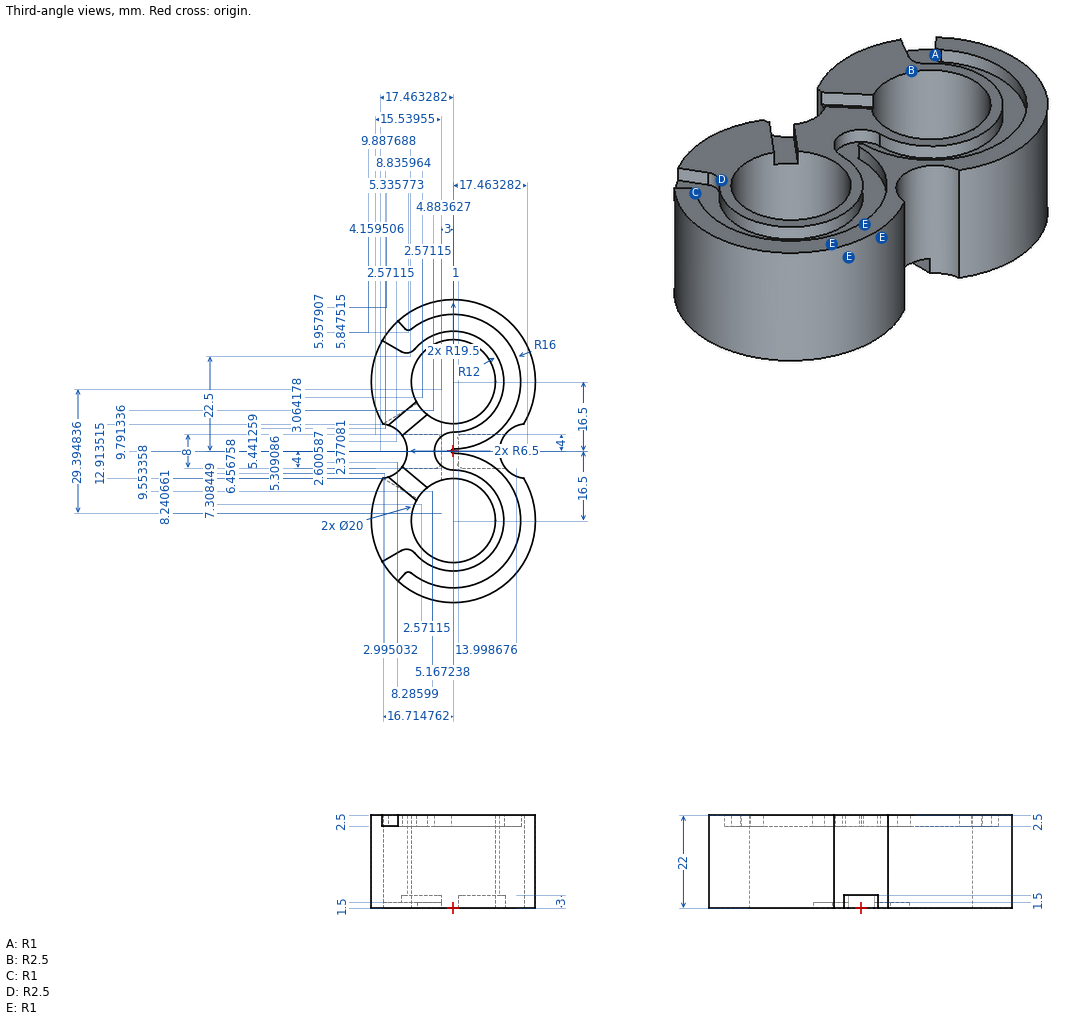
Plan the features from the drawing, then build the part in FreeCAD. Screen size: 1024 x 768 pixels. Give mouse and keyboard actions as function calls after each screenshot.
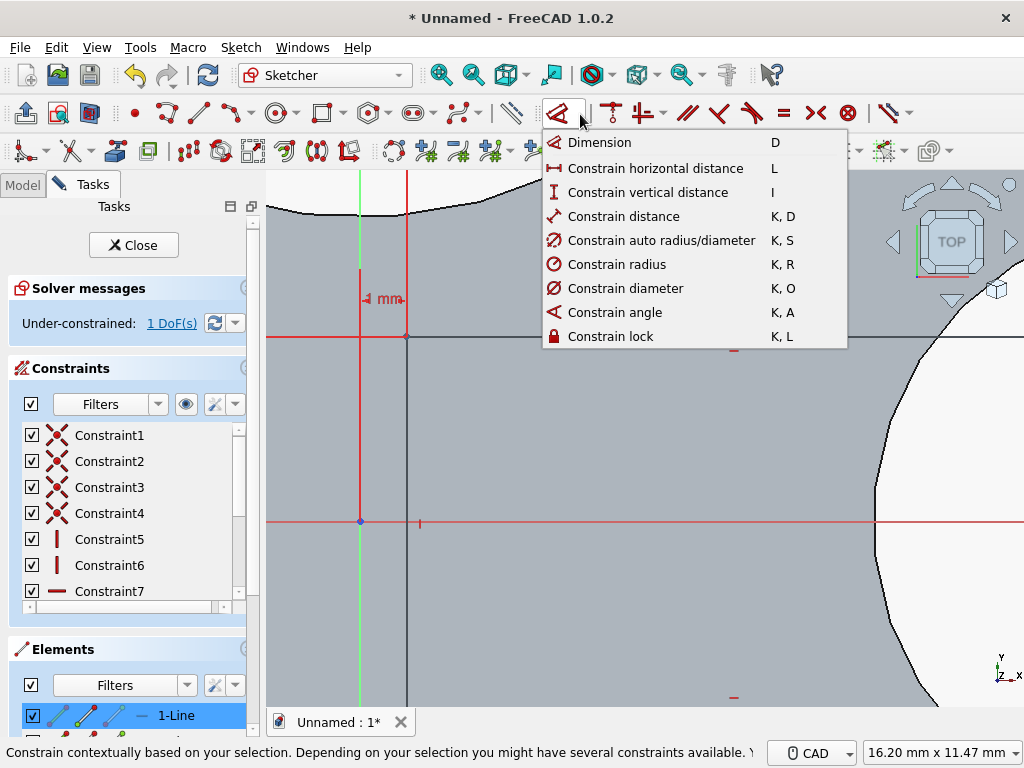
click(695, 192)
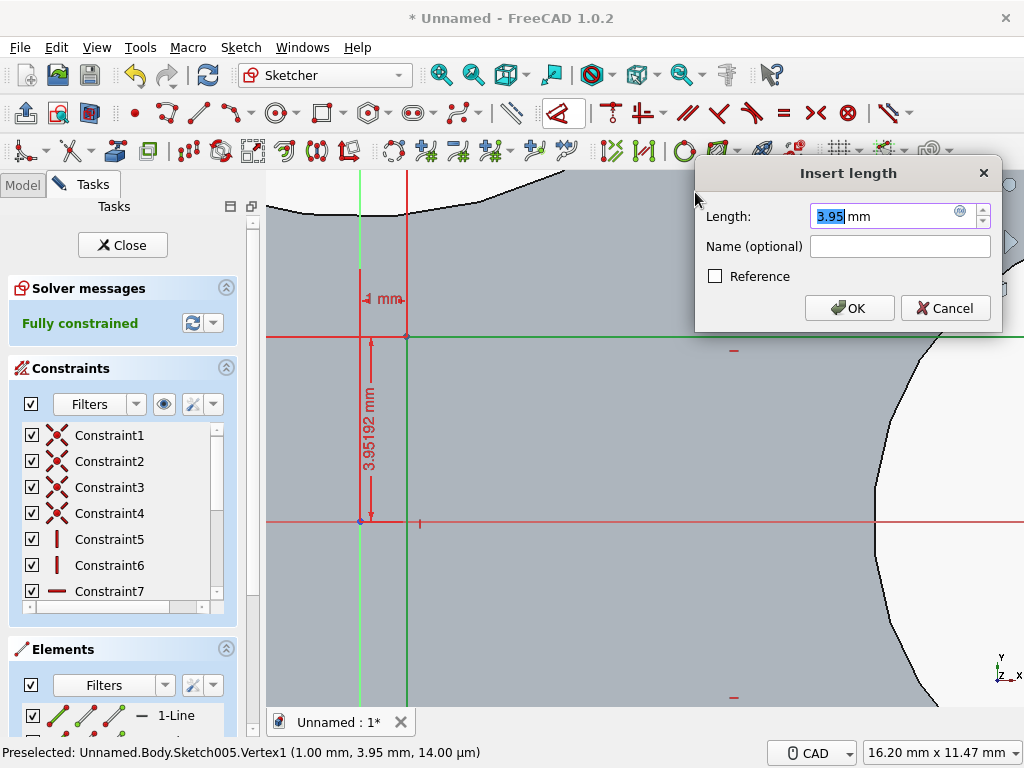
text(4)
key(Return)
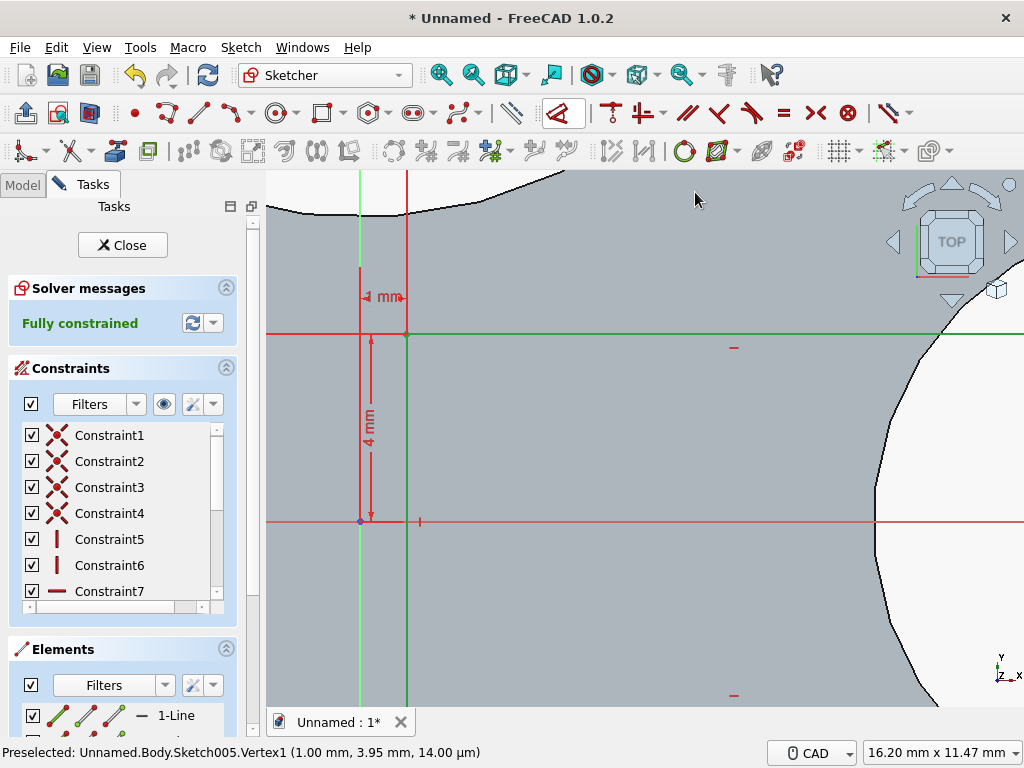
click(123, 245)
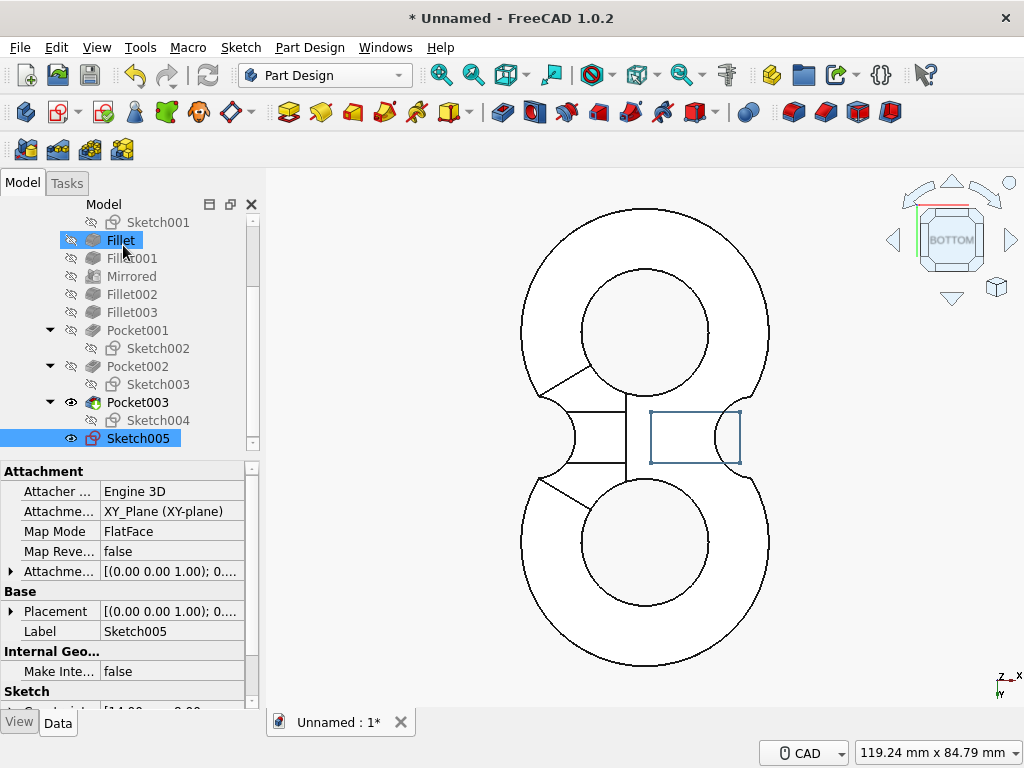
click(504, 112)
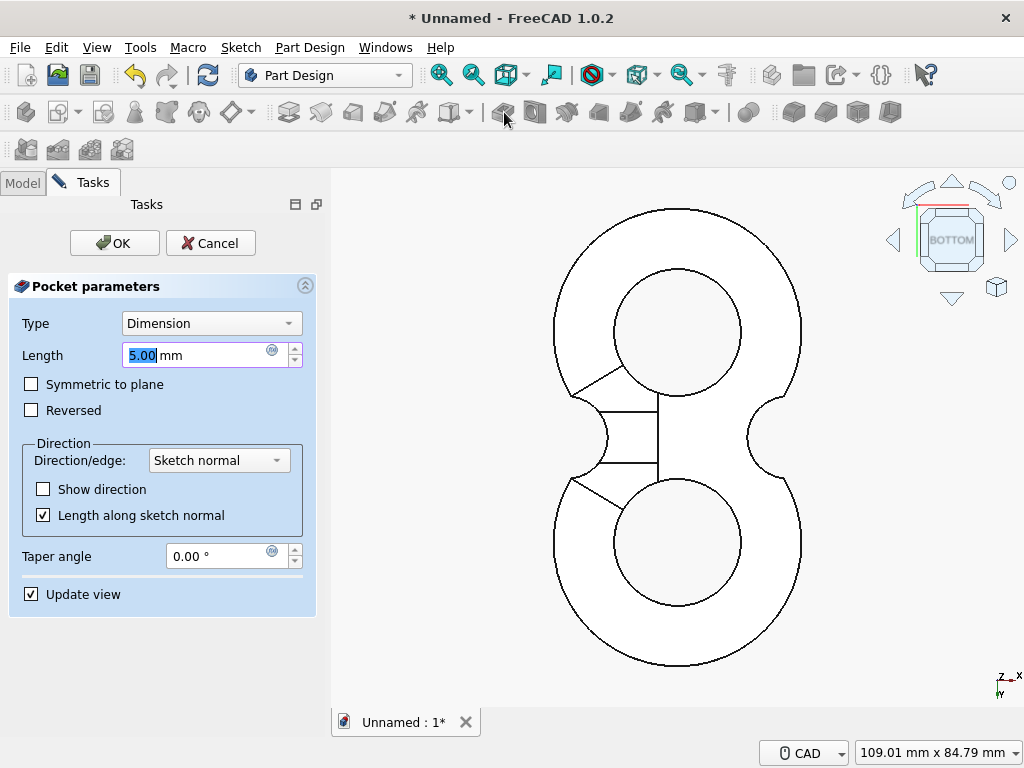
text(3)
key(Tab)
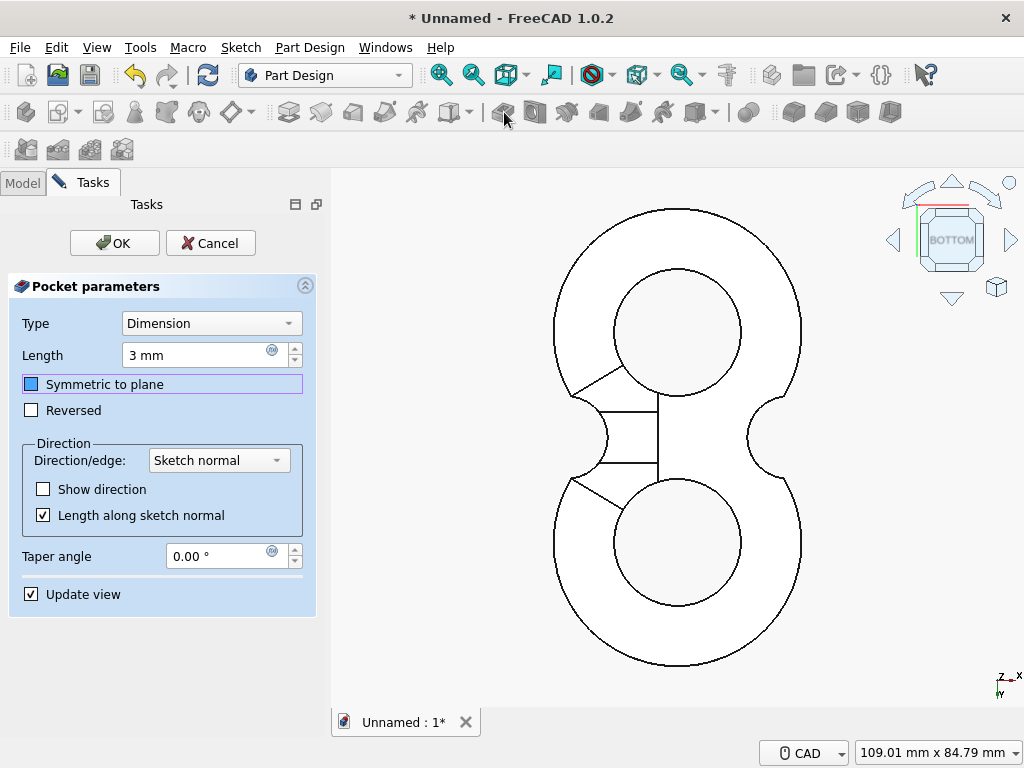
click(30, 410)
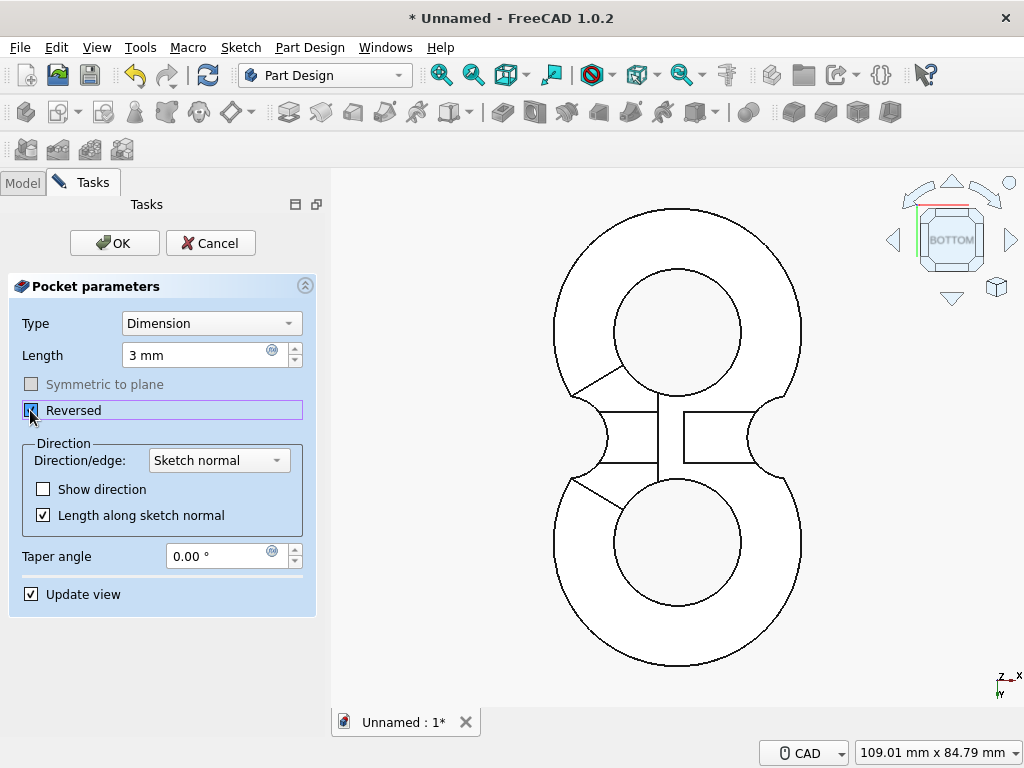
click(115, 243)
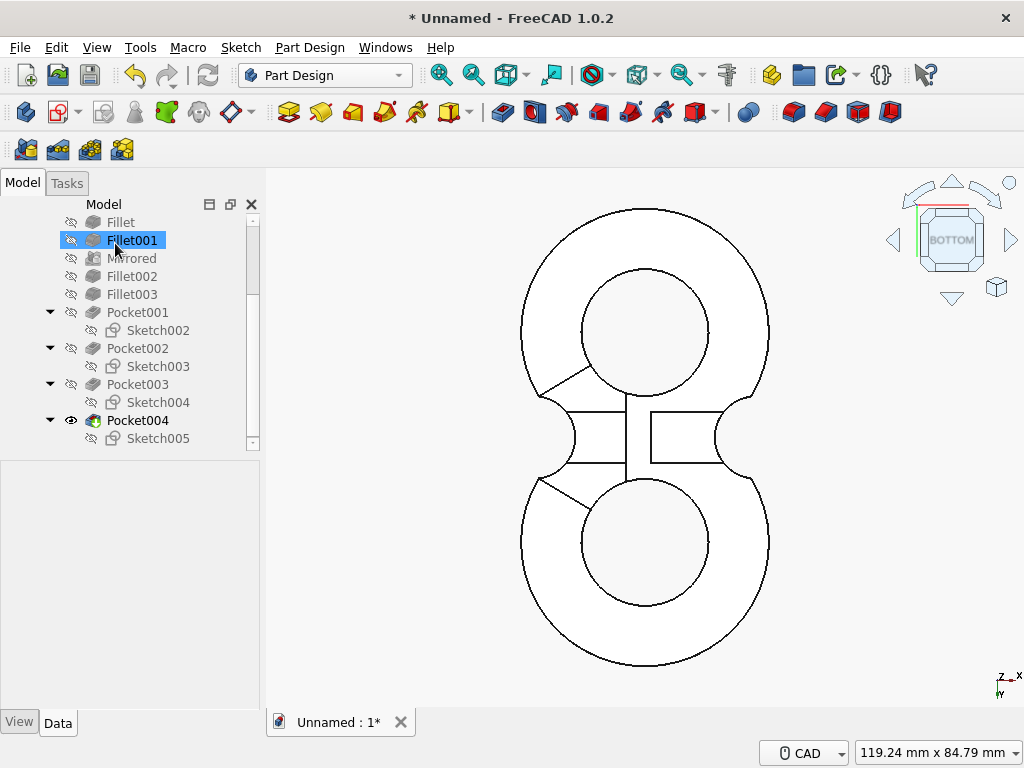
scroll(626, 462, up, 8)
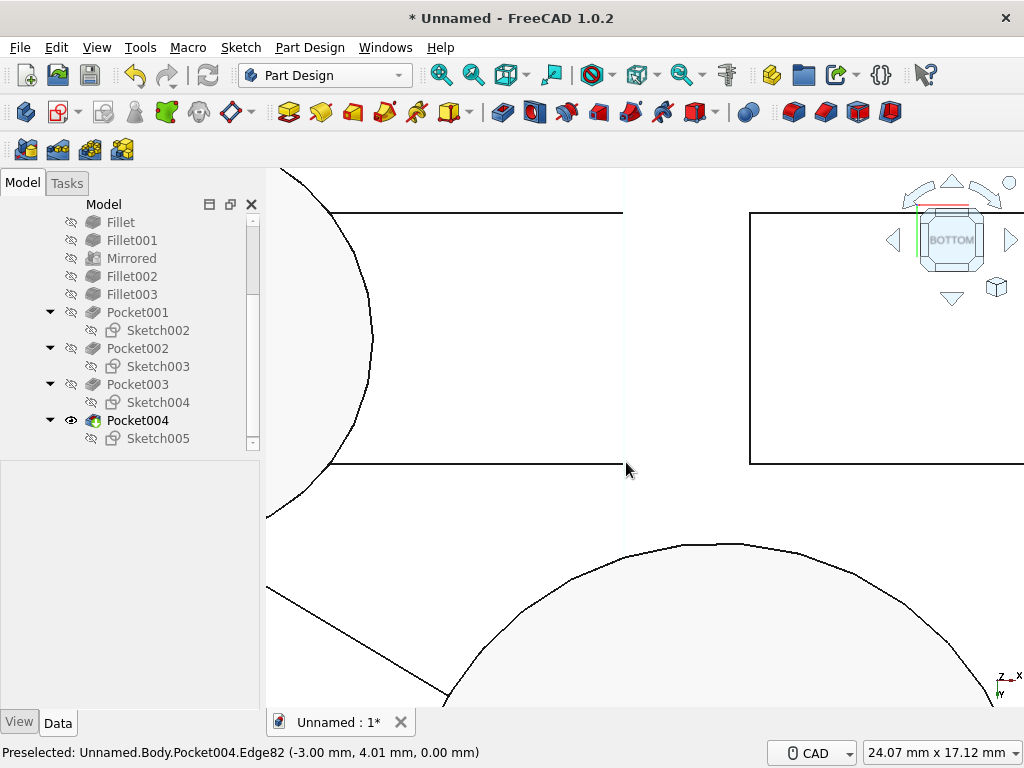
key(v)
key(f)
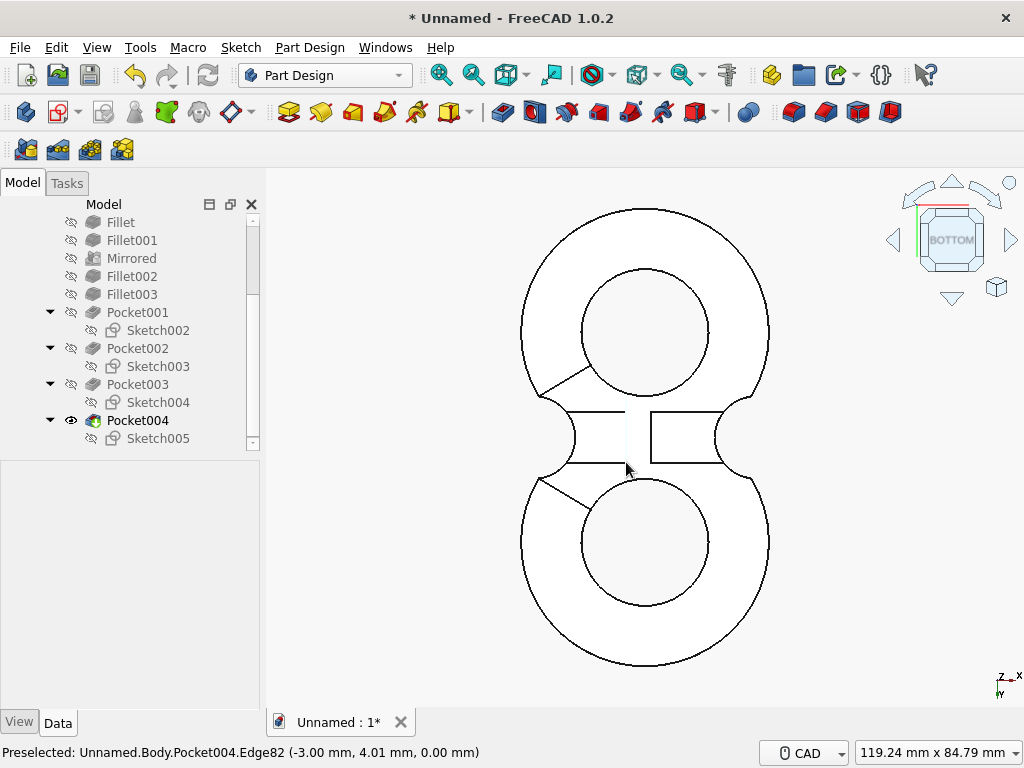
key(0)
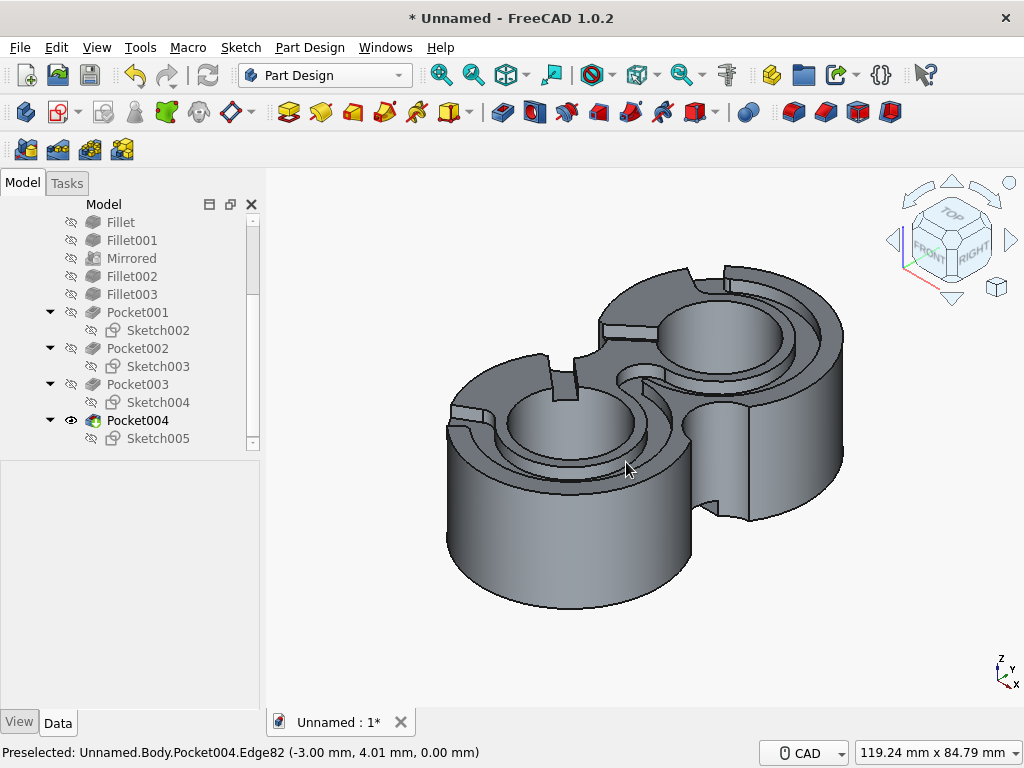
scroll(649, 464, up, 8)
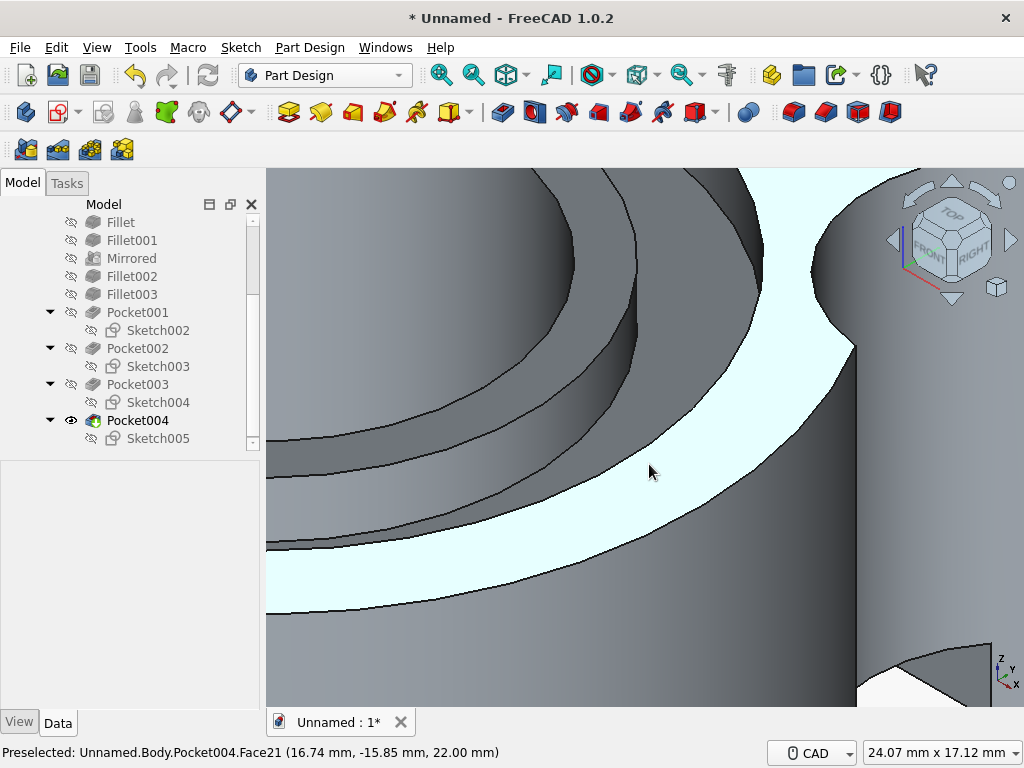
key(v)
key(f)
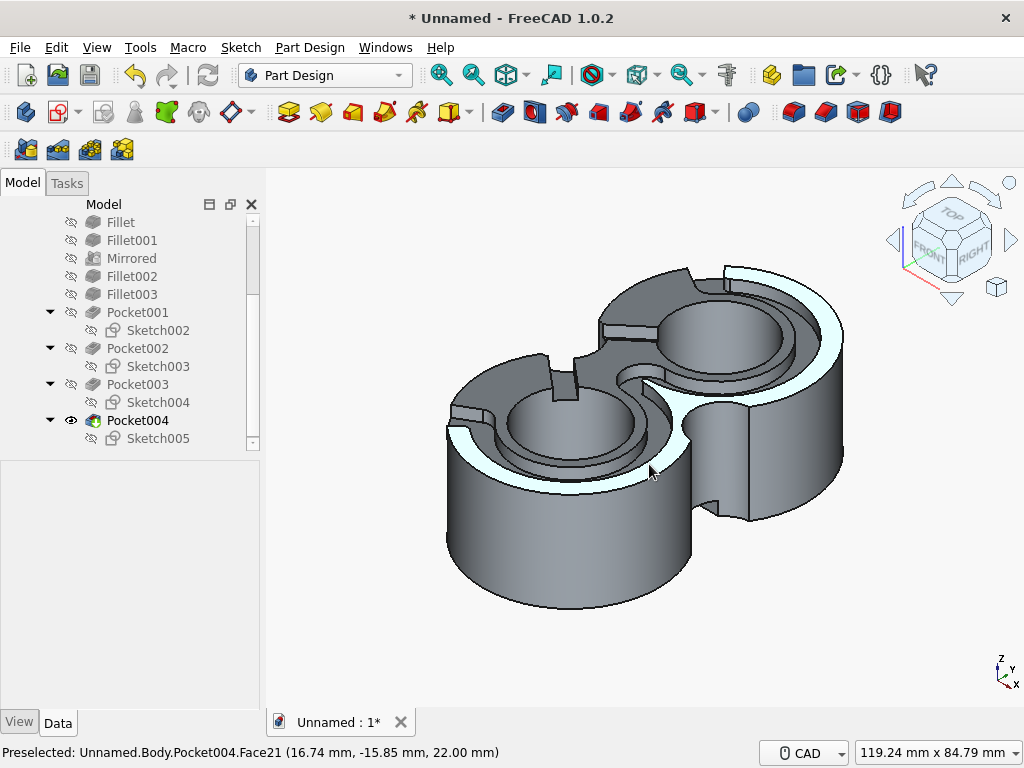
key(2)